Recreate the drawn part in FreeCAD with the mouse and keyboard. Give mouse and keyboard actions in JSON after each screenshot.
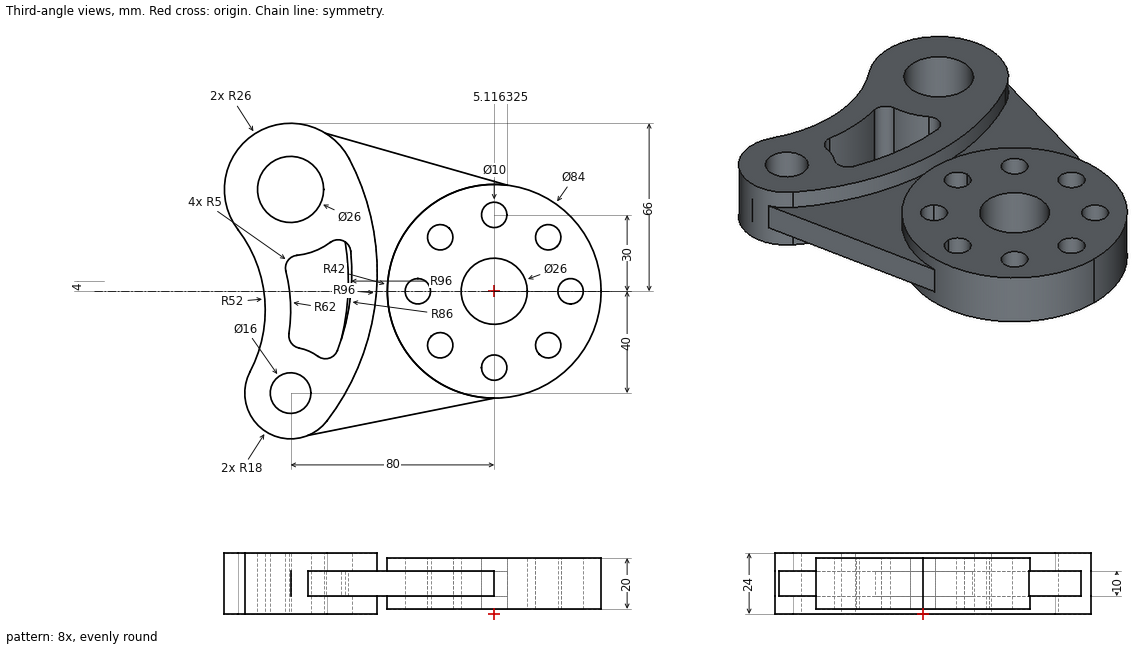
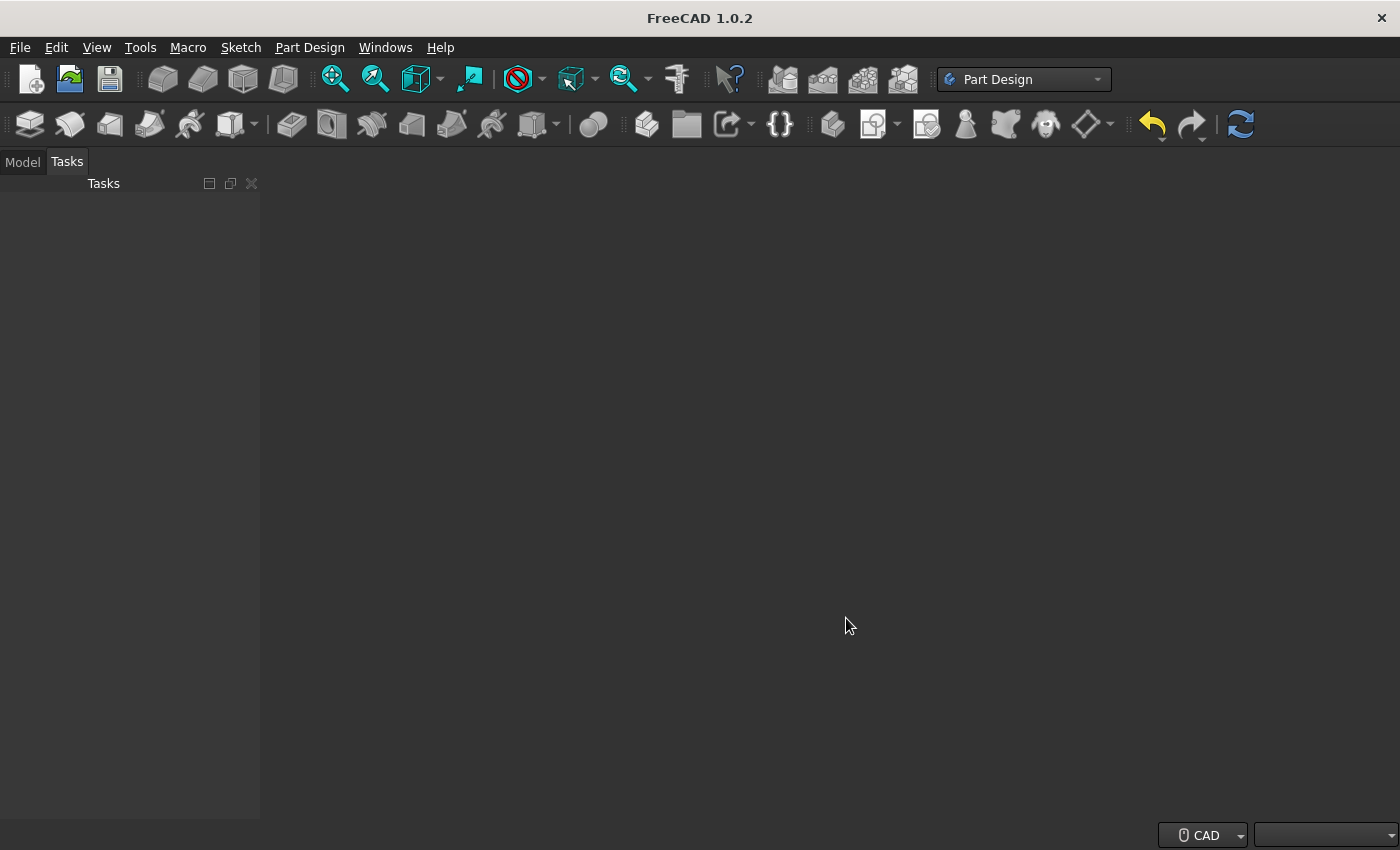
{"action": "left_click", "coordinate": [30, 80]}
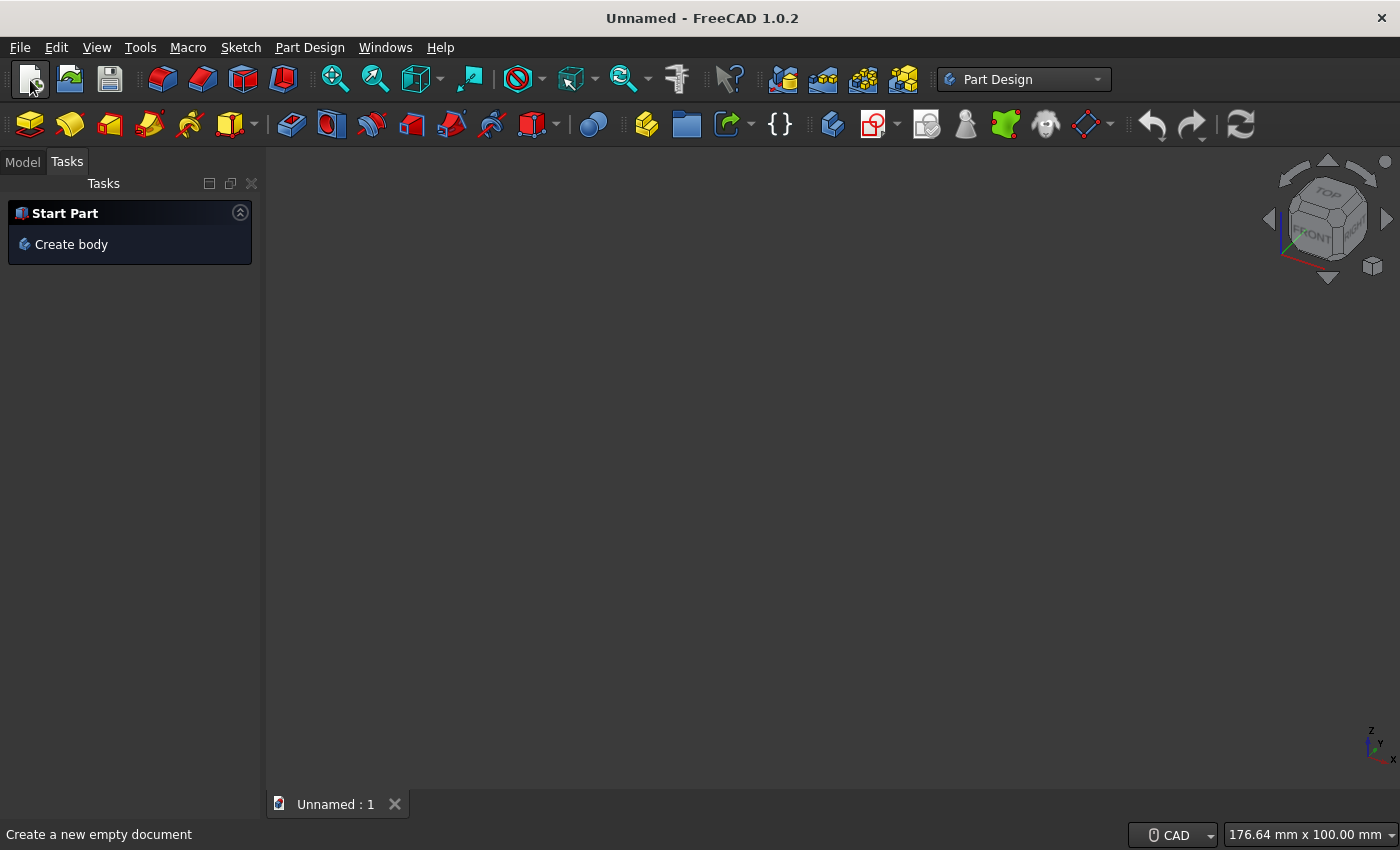
{"action": "left_click", "coordinate": [874, 124]}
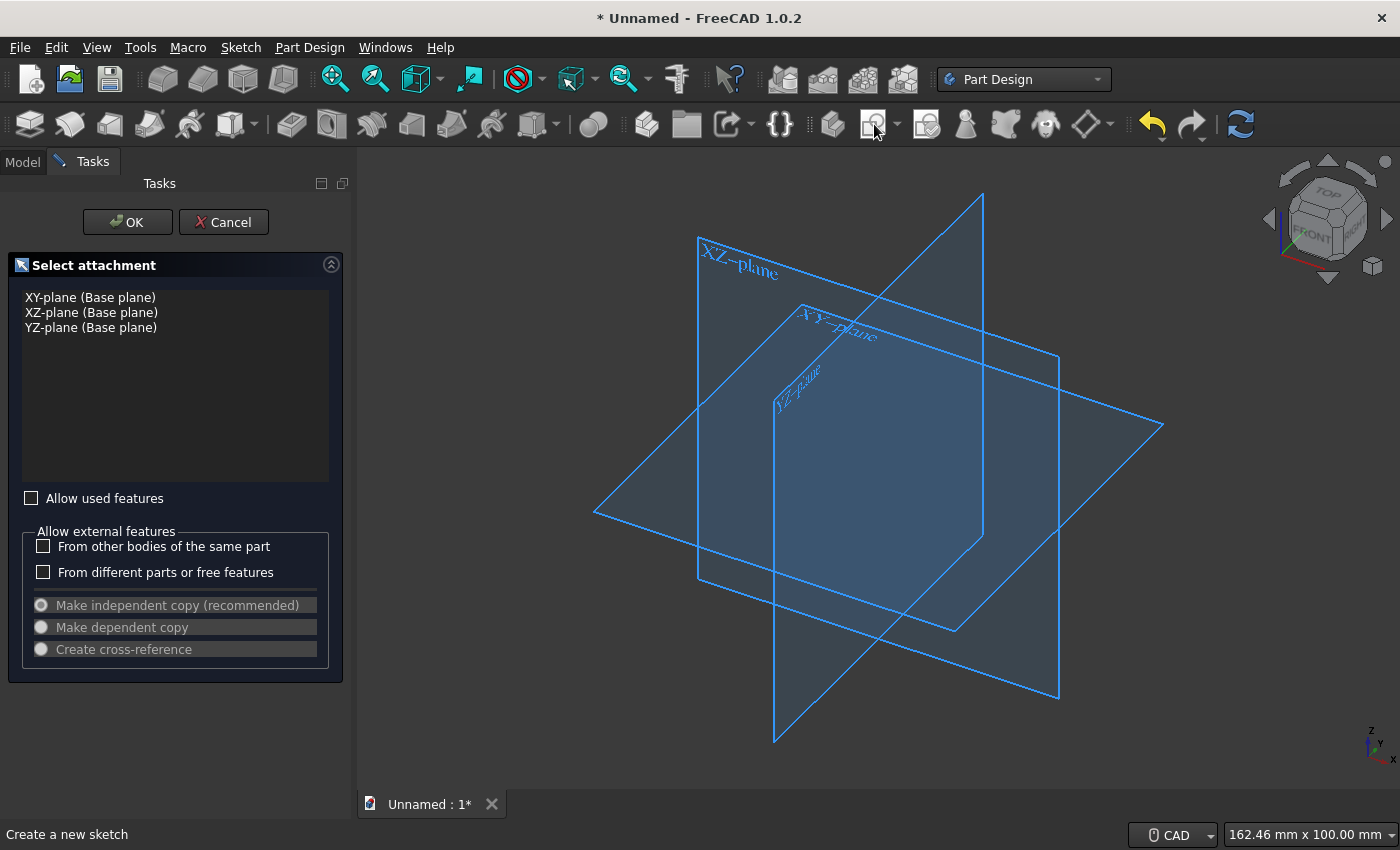
{"action": "left_click", "coordinate": [82, 298]}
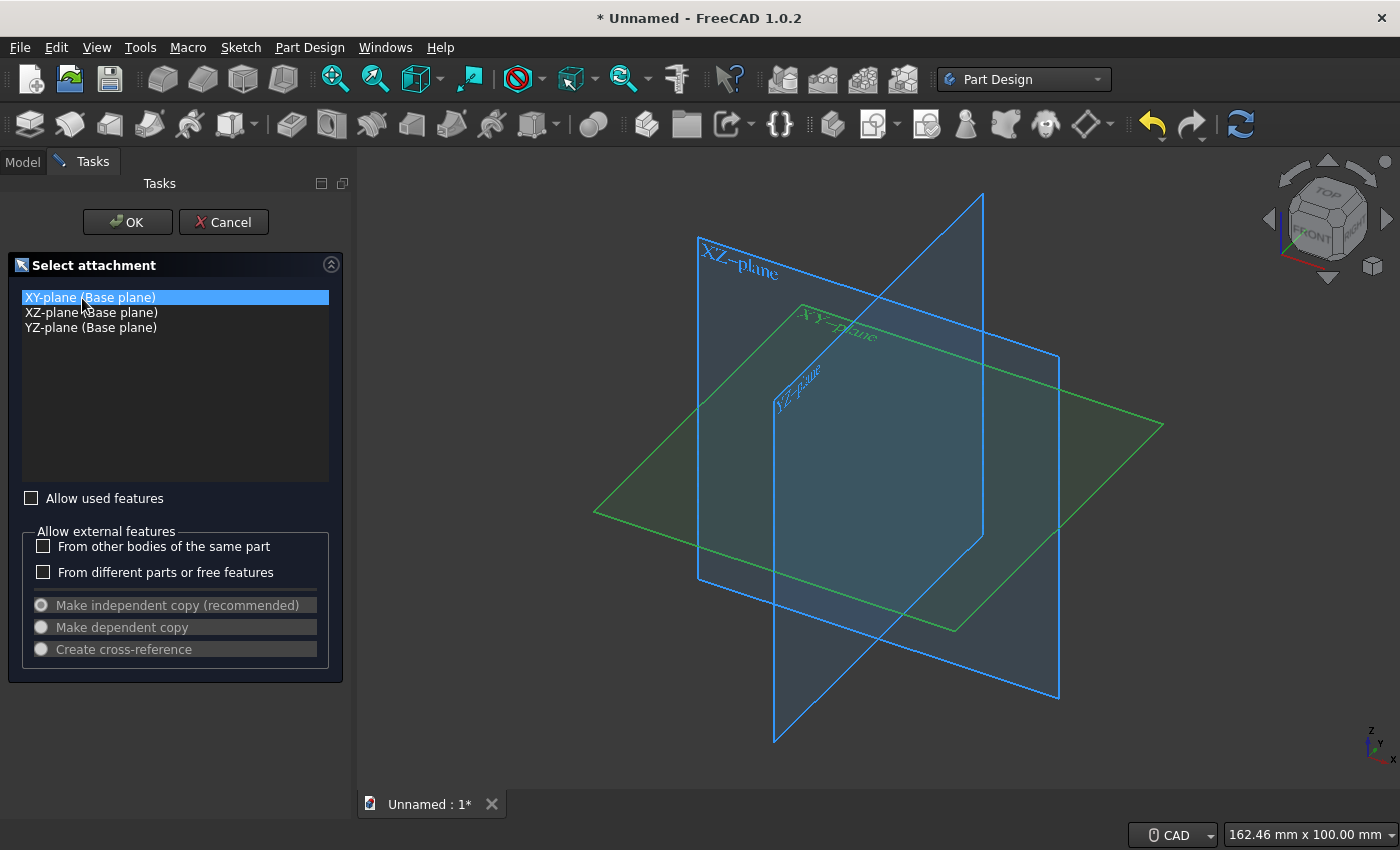
{"action": "left_click", "coordinate": [128, 222]}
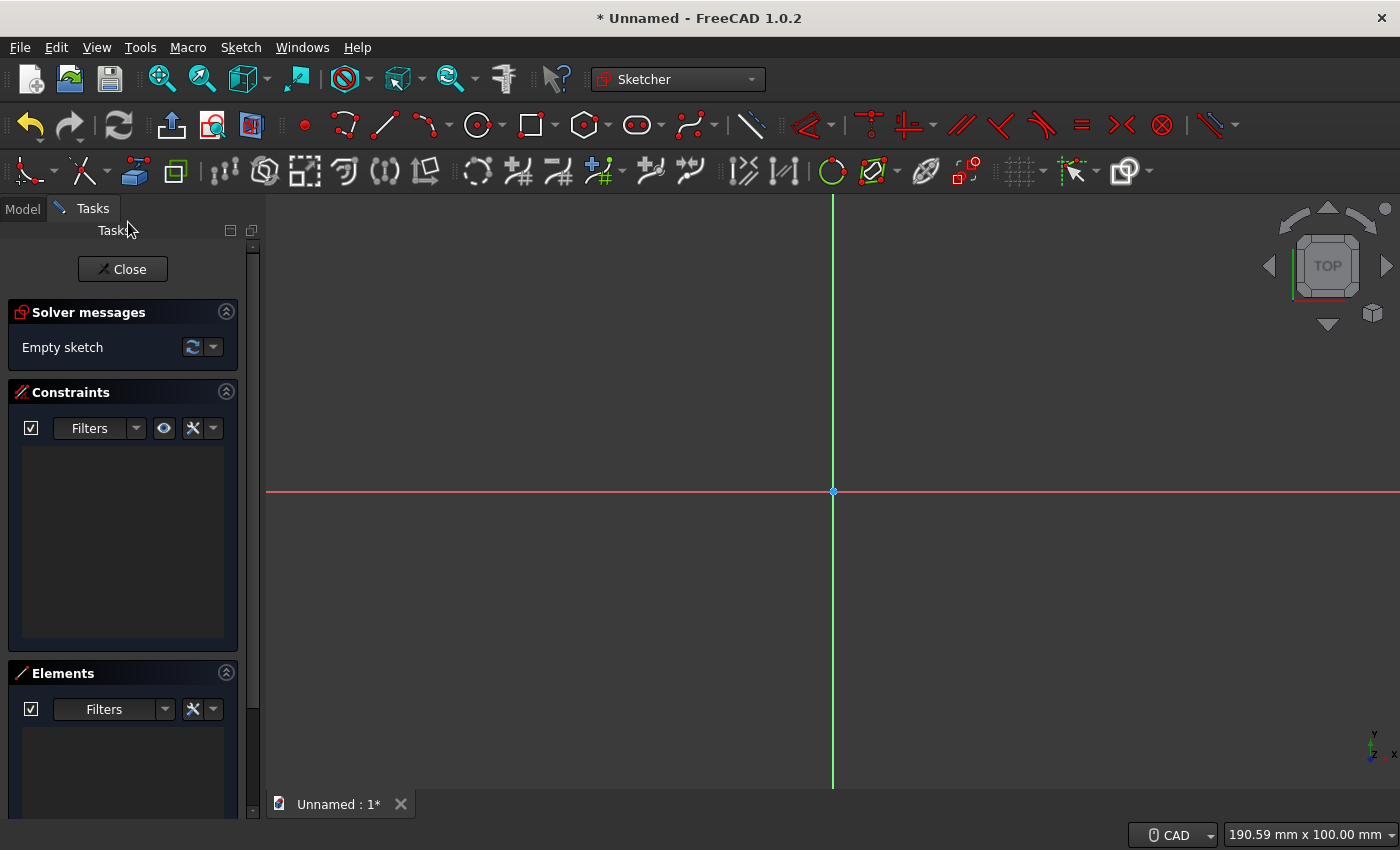
{"action": "scroll", "coordinate": [1045, 516], "scroll_direction": "down", "scroll_amount": 3}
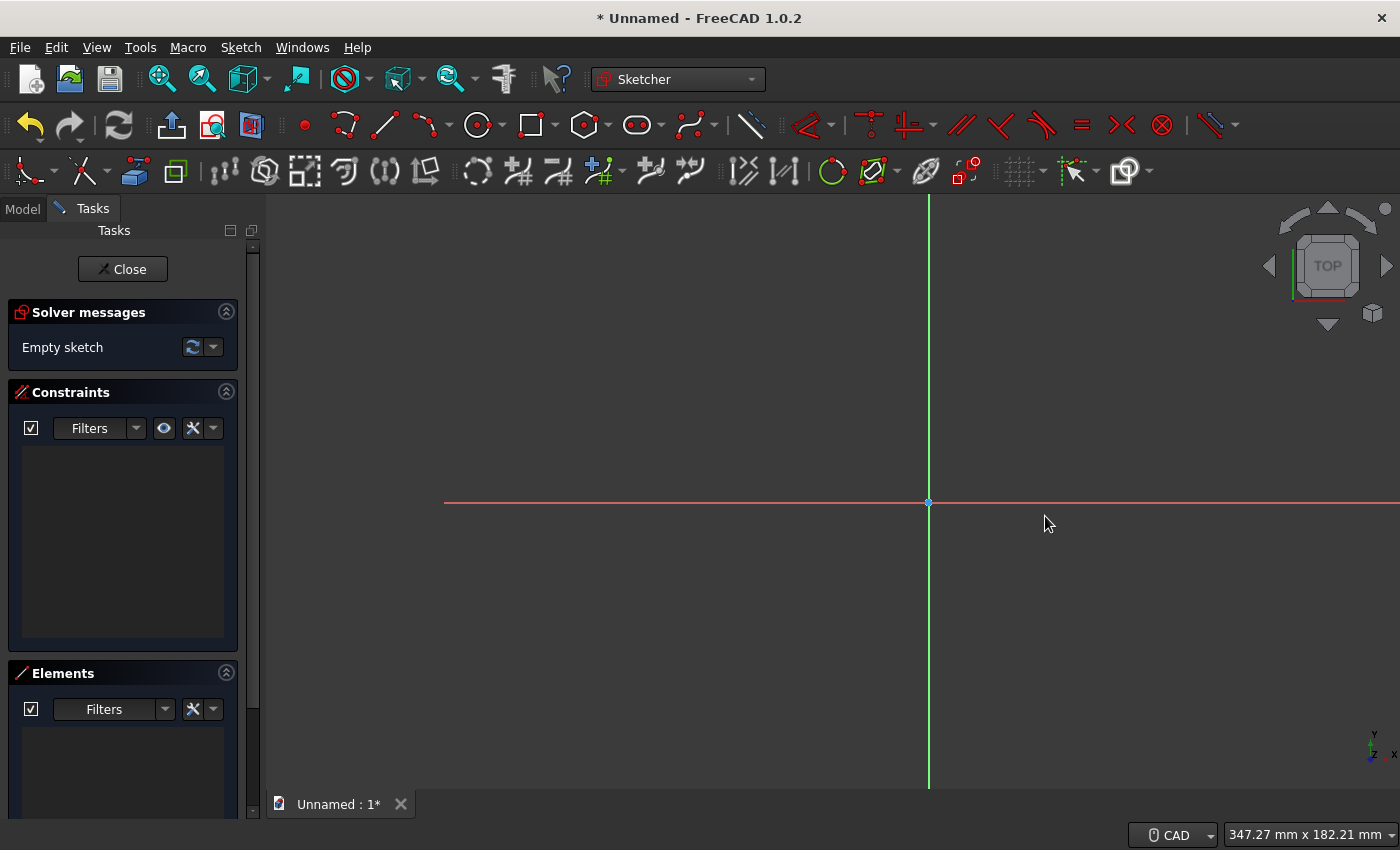
{"action": "left_click", "coordinate": [426, 126]}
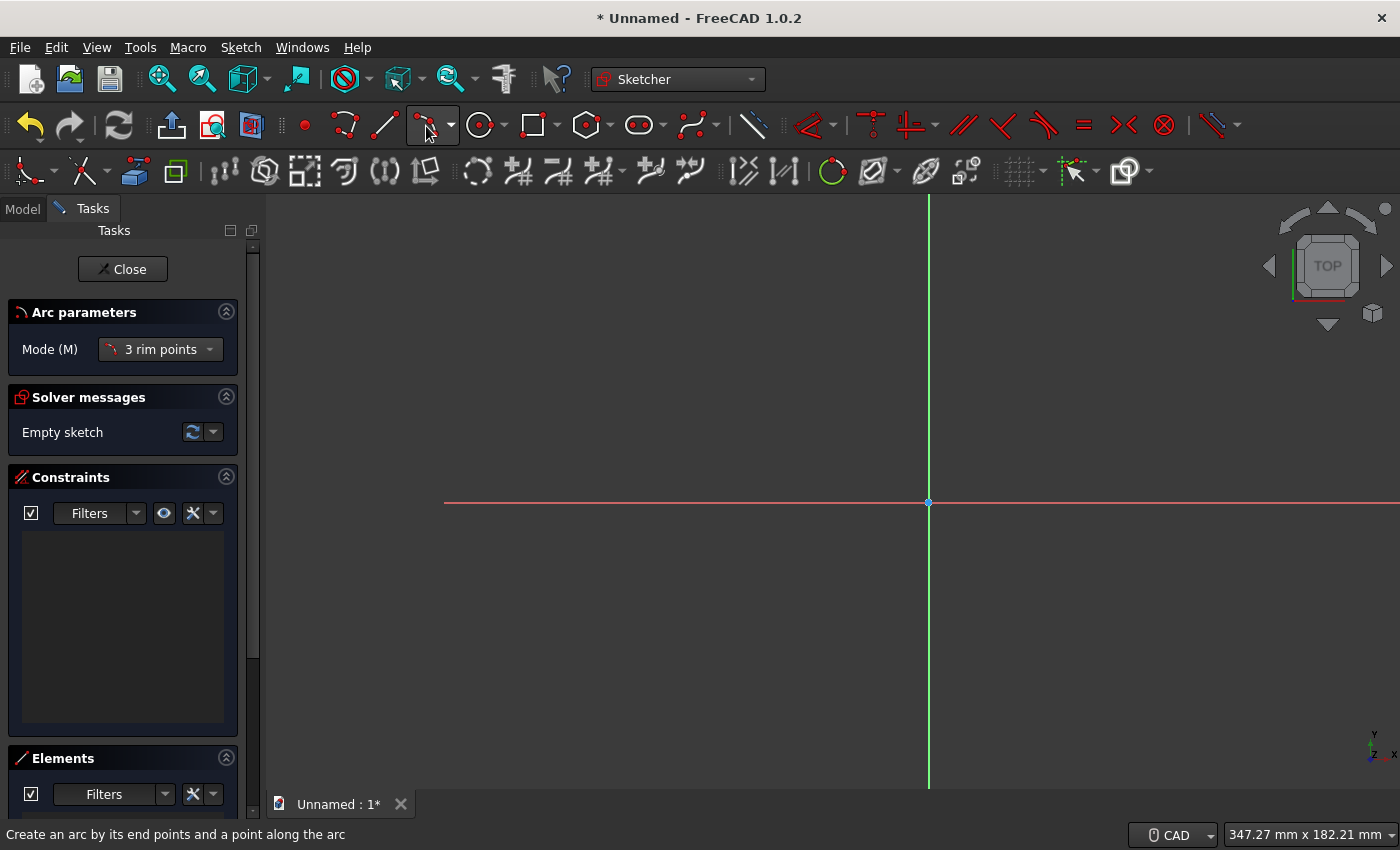
{"action": "left_click", "coordinate": [743, 333]}
{"action": "left_click", "coordinate": [600, 424]}
{"action": "left_click", "coordinate": [622, 301]}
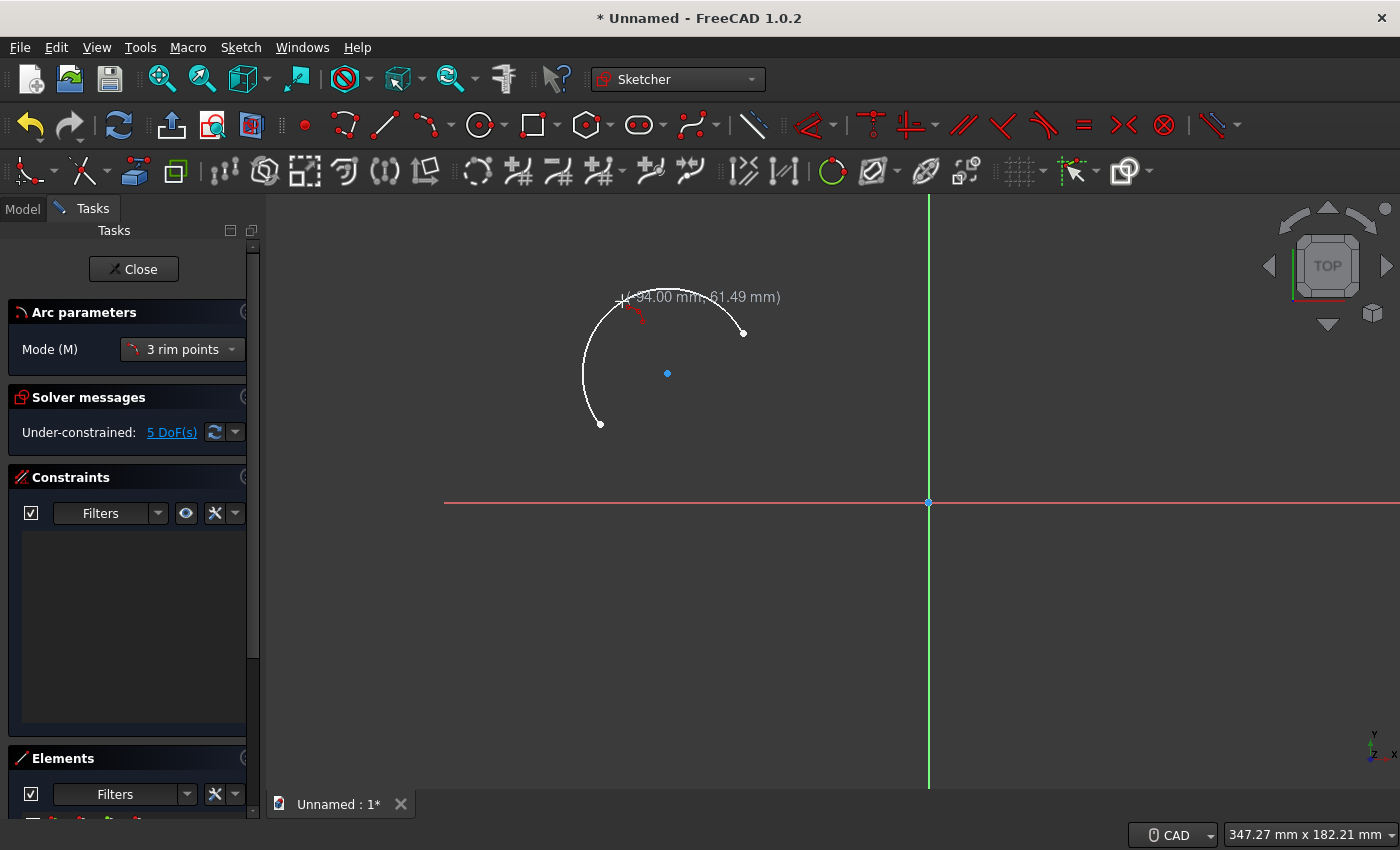
{"action": "left_click", "coordinate": [600, 425]}
{"action": "left_click", "coordinate": [616, 606]}
{"action": "left_click", "coordinate": [635, 532]}